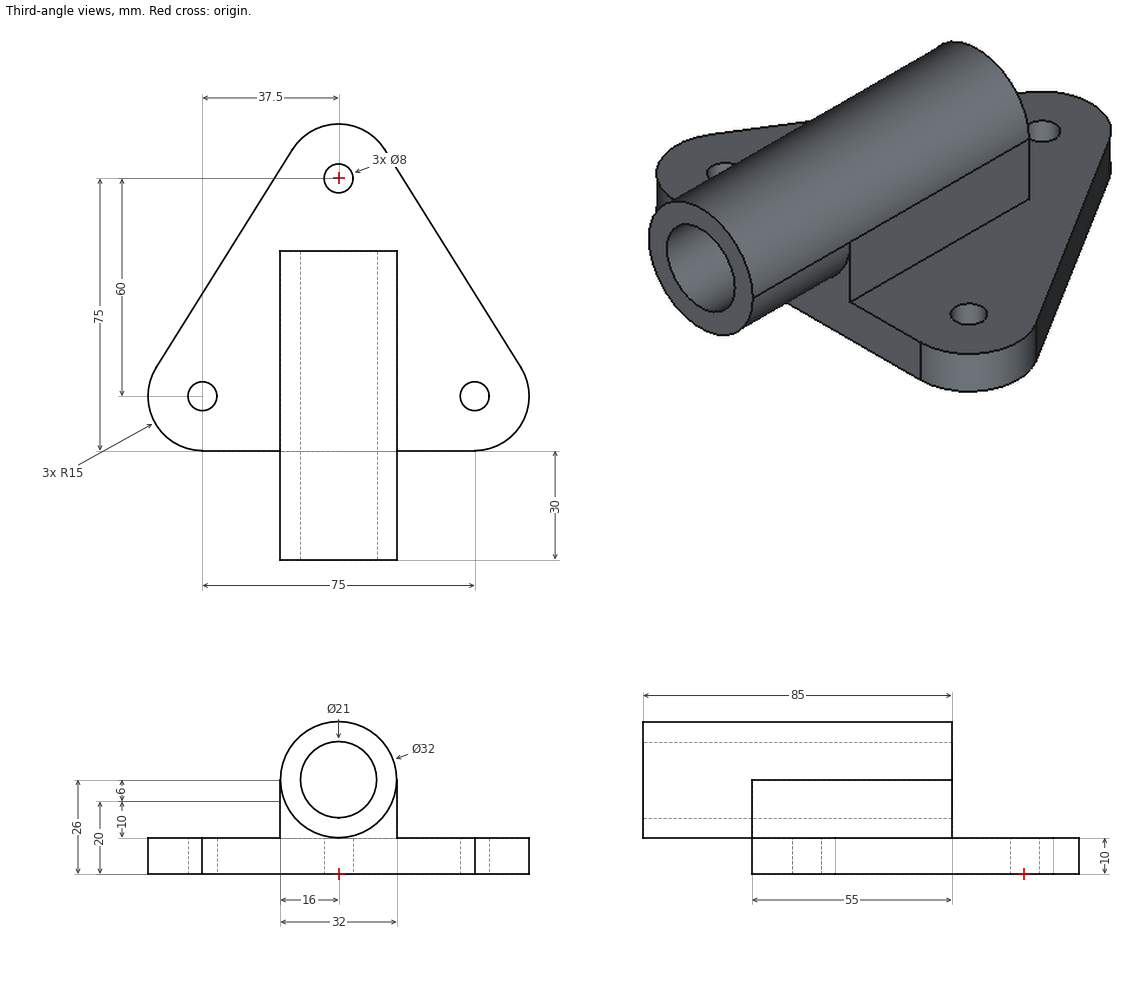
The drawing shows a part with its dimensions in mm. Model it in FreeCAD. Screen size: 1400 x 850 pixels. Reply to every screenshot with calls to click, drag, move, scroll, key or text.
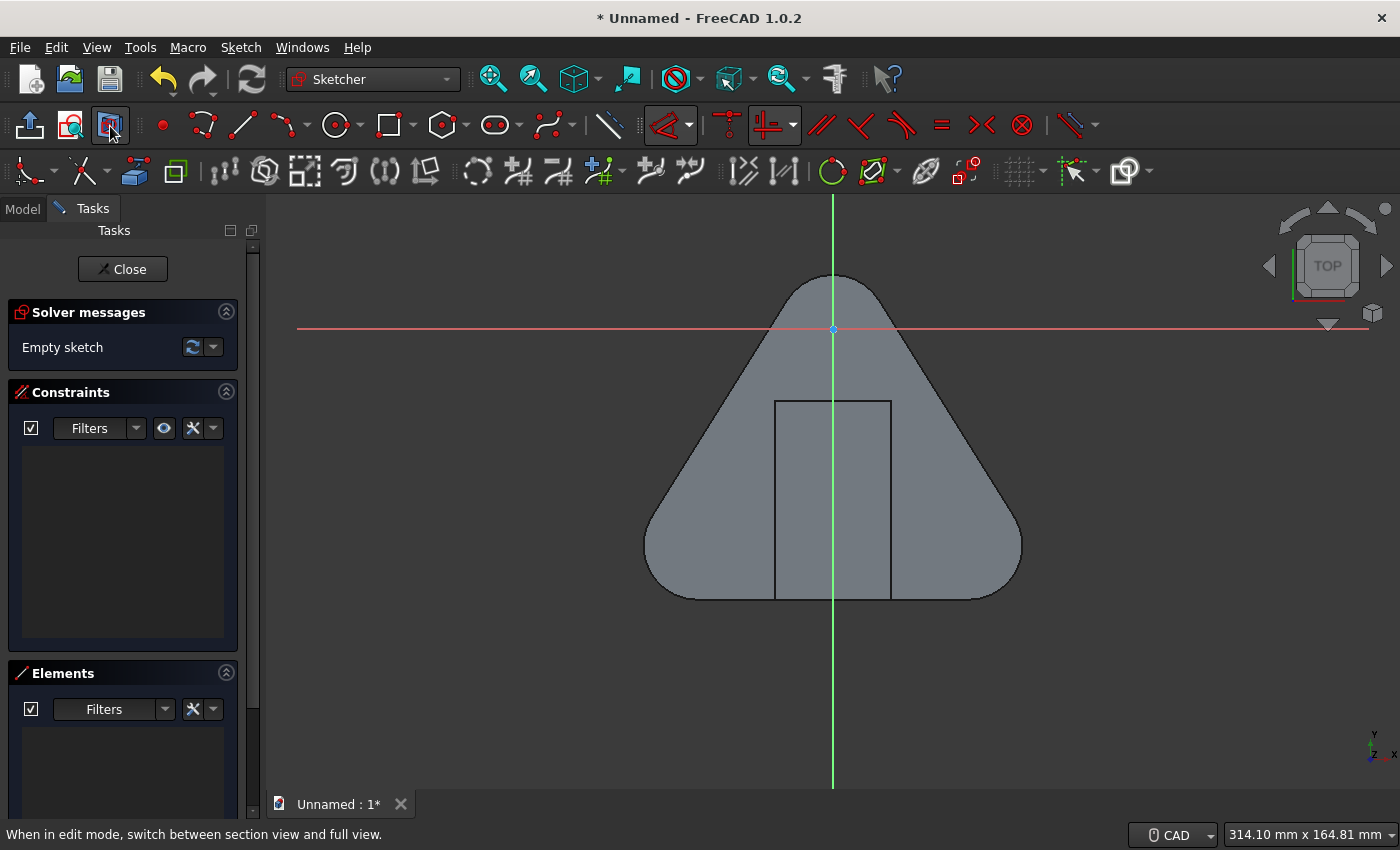
scroll(972, 327, up, 2)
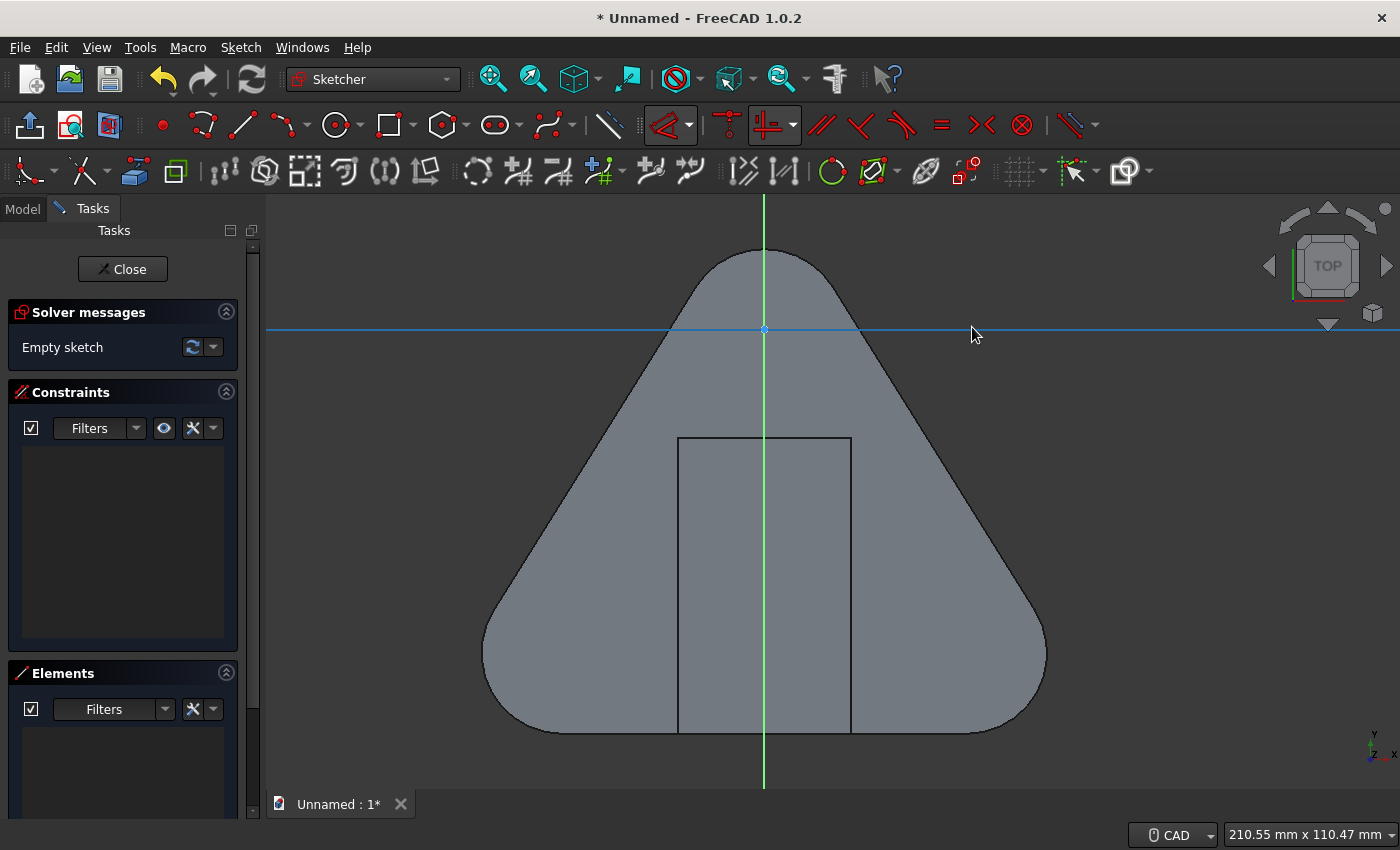
click(336, 126)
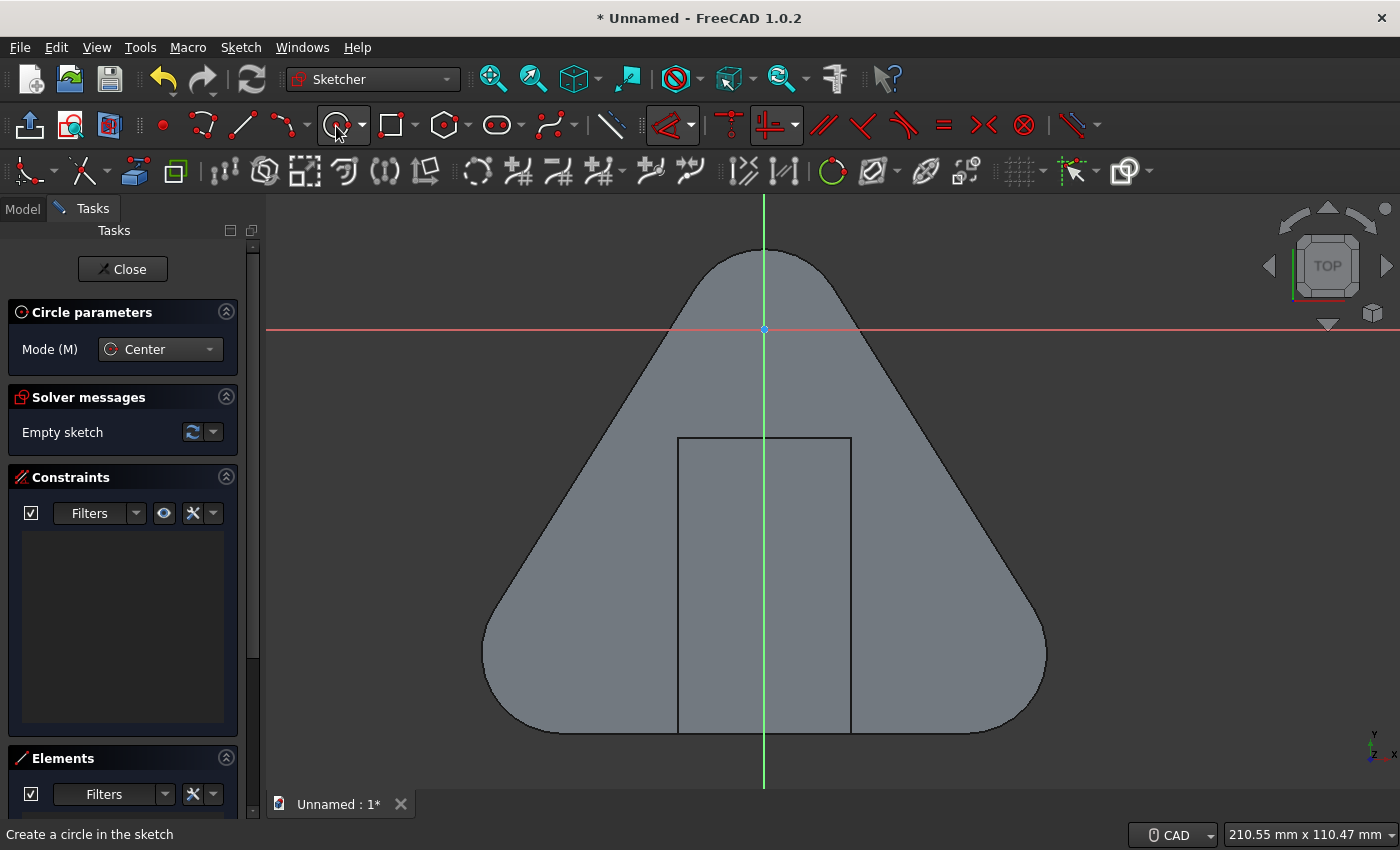
click(764, 330)
click(780, 315)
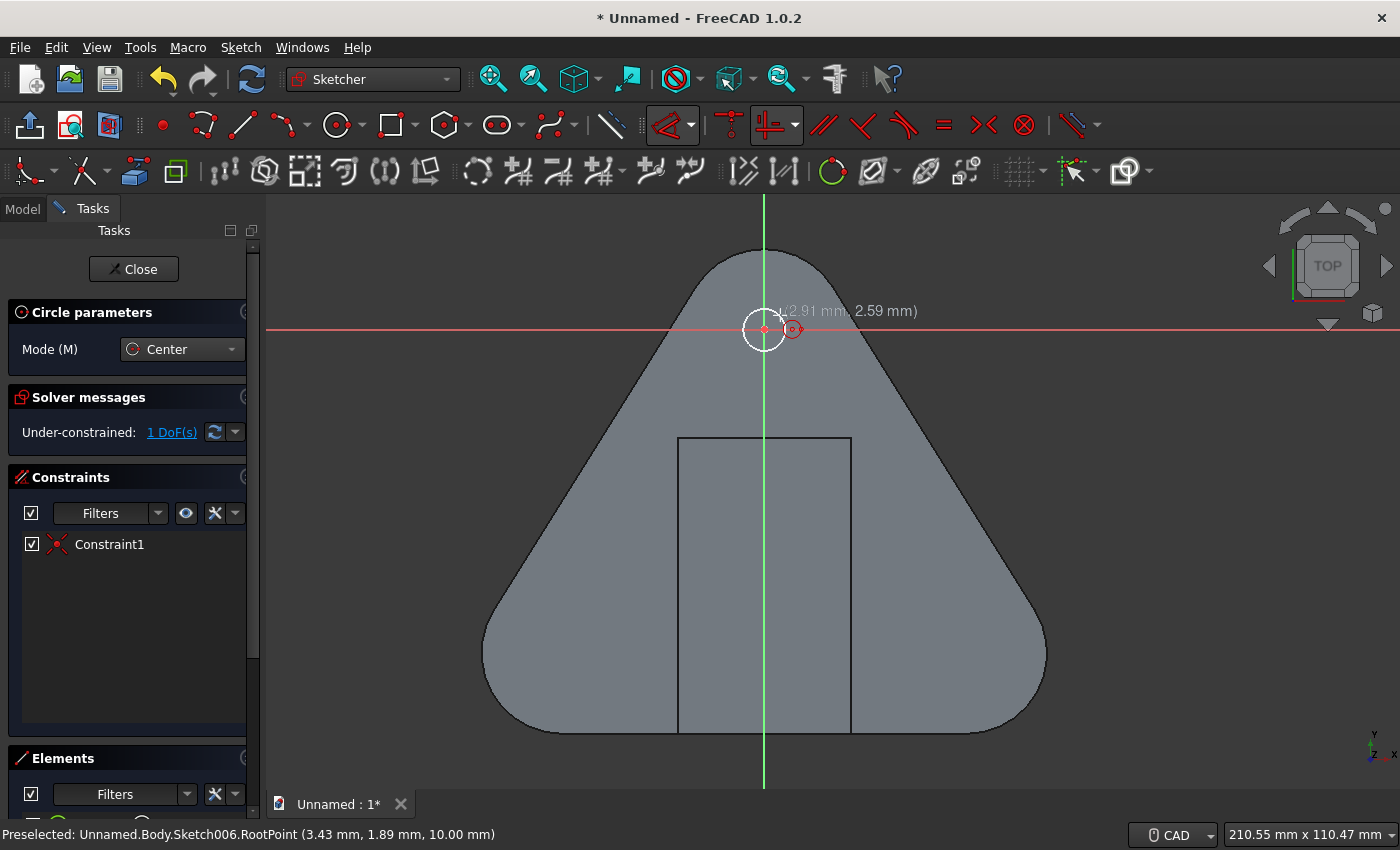
click(562, 653)
click(578, 638)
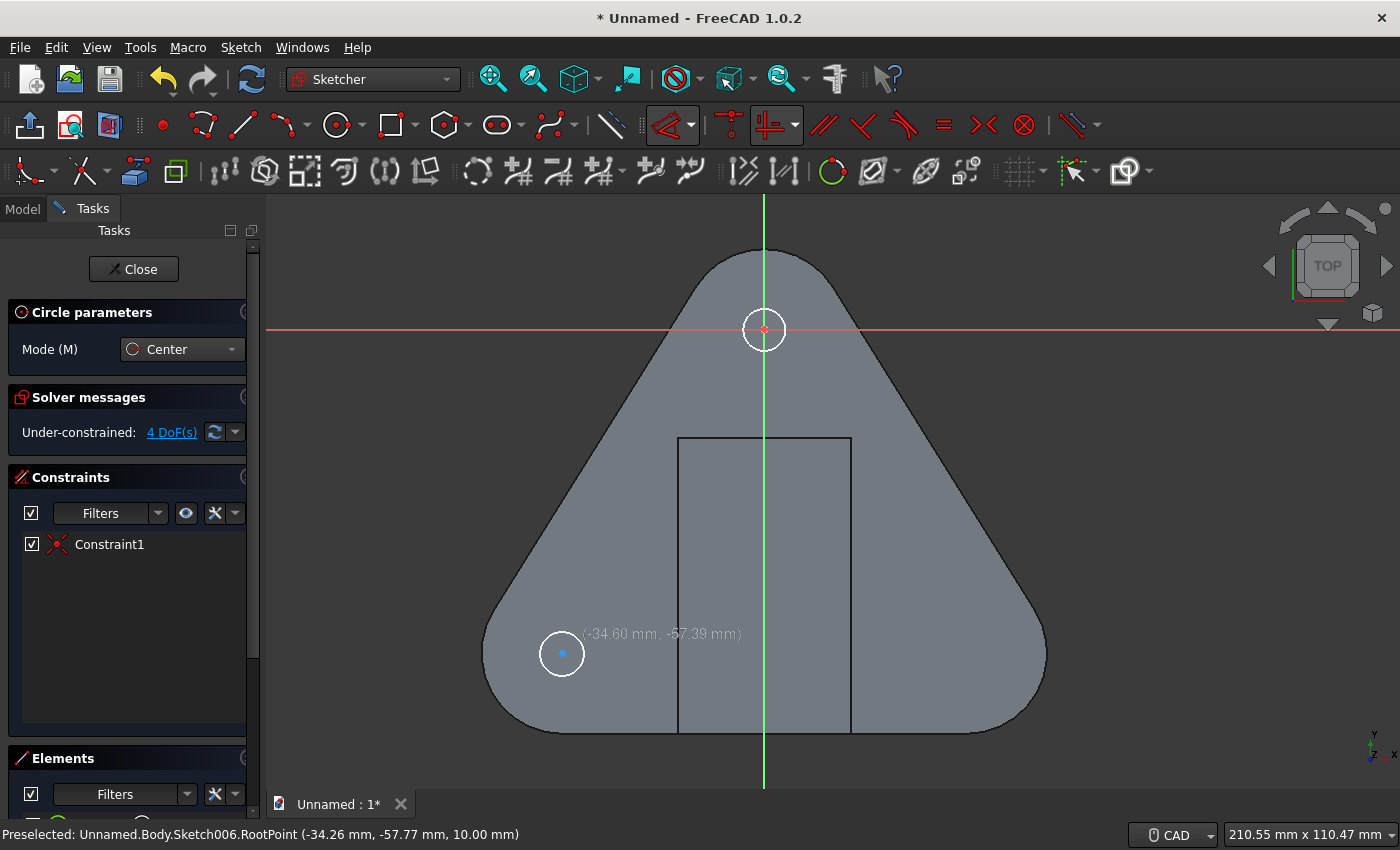
click(966, 653)
click(982, 638)
key(Escape)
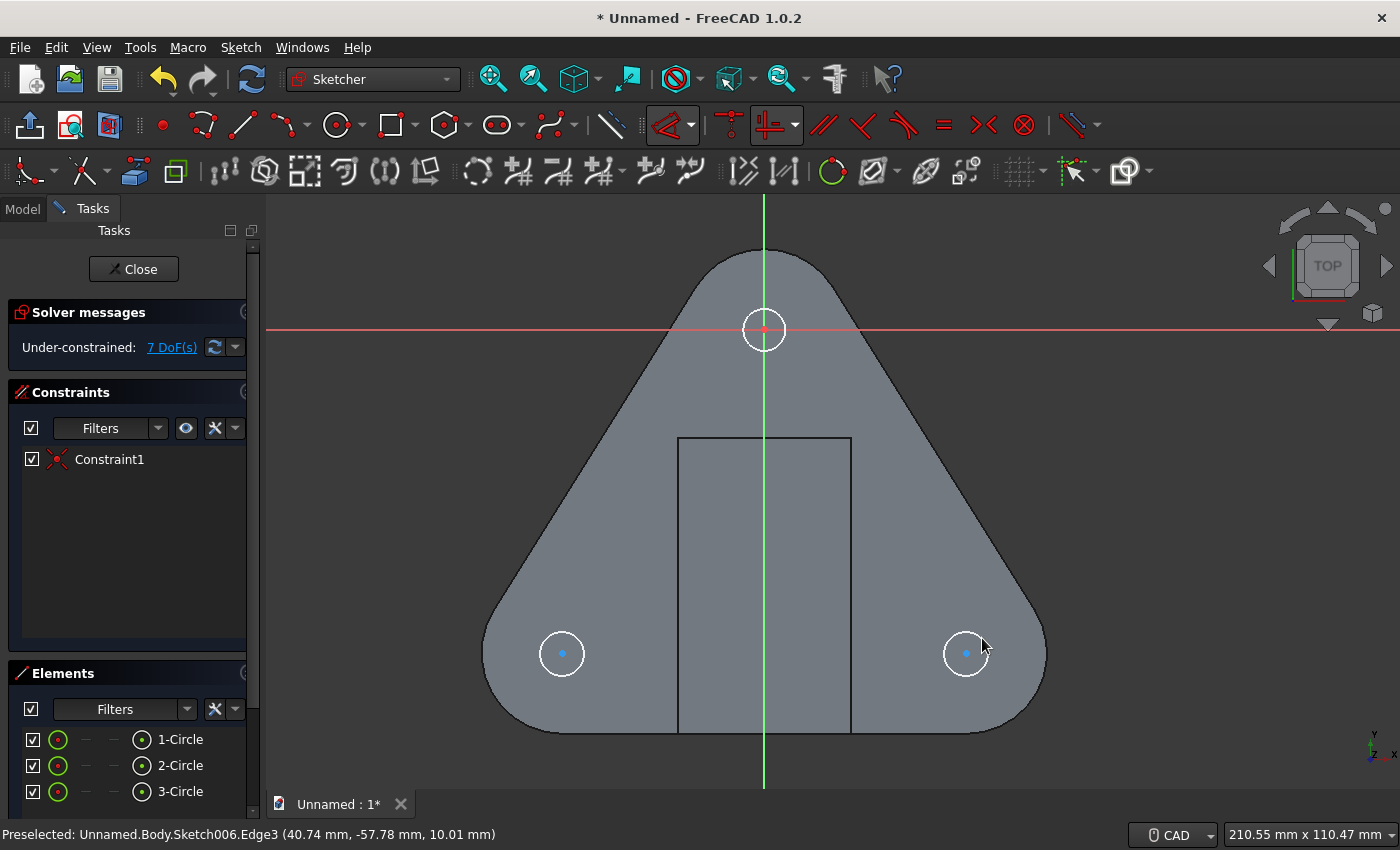
click(779, 315)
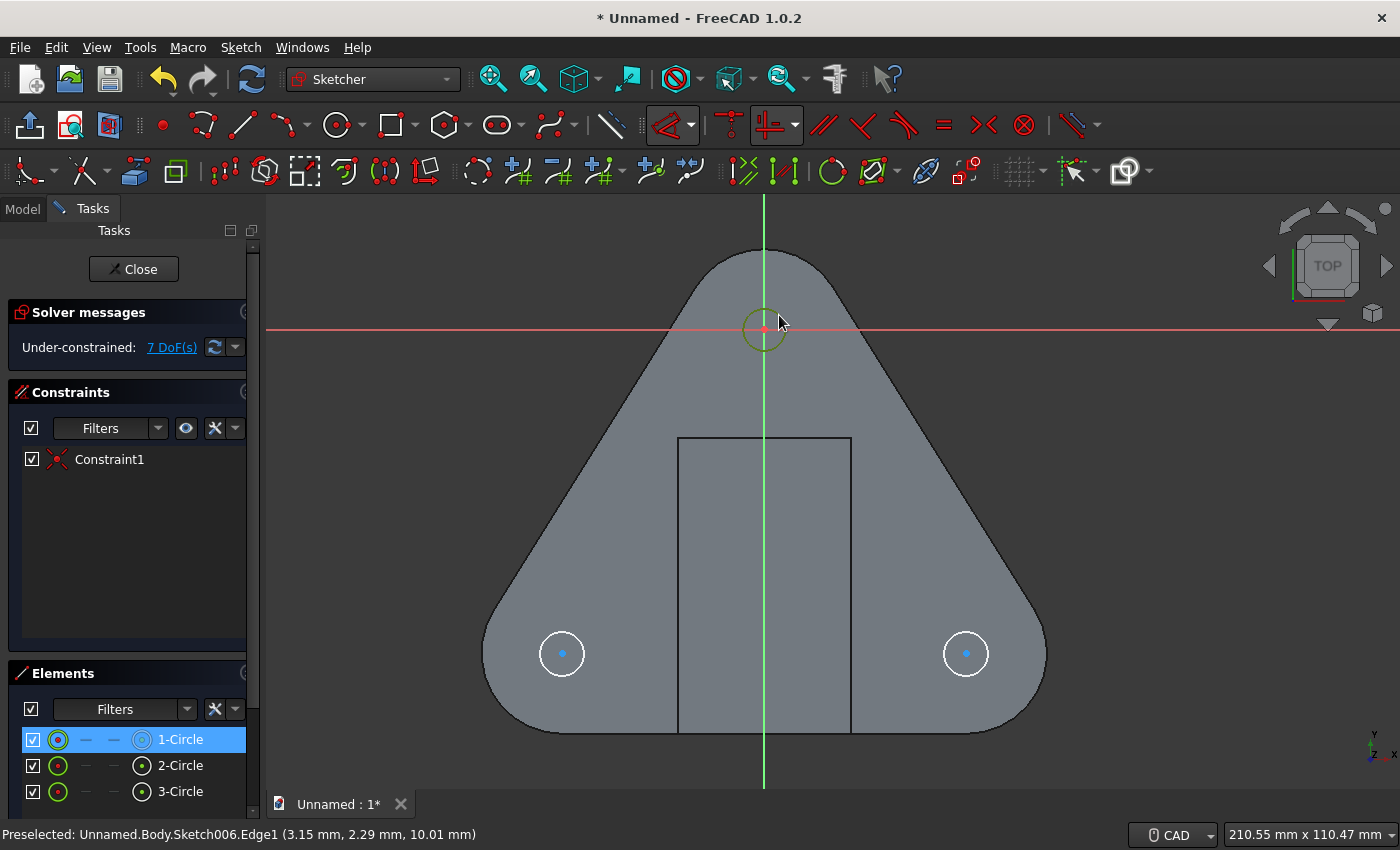
click(577, 638)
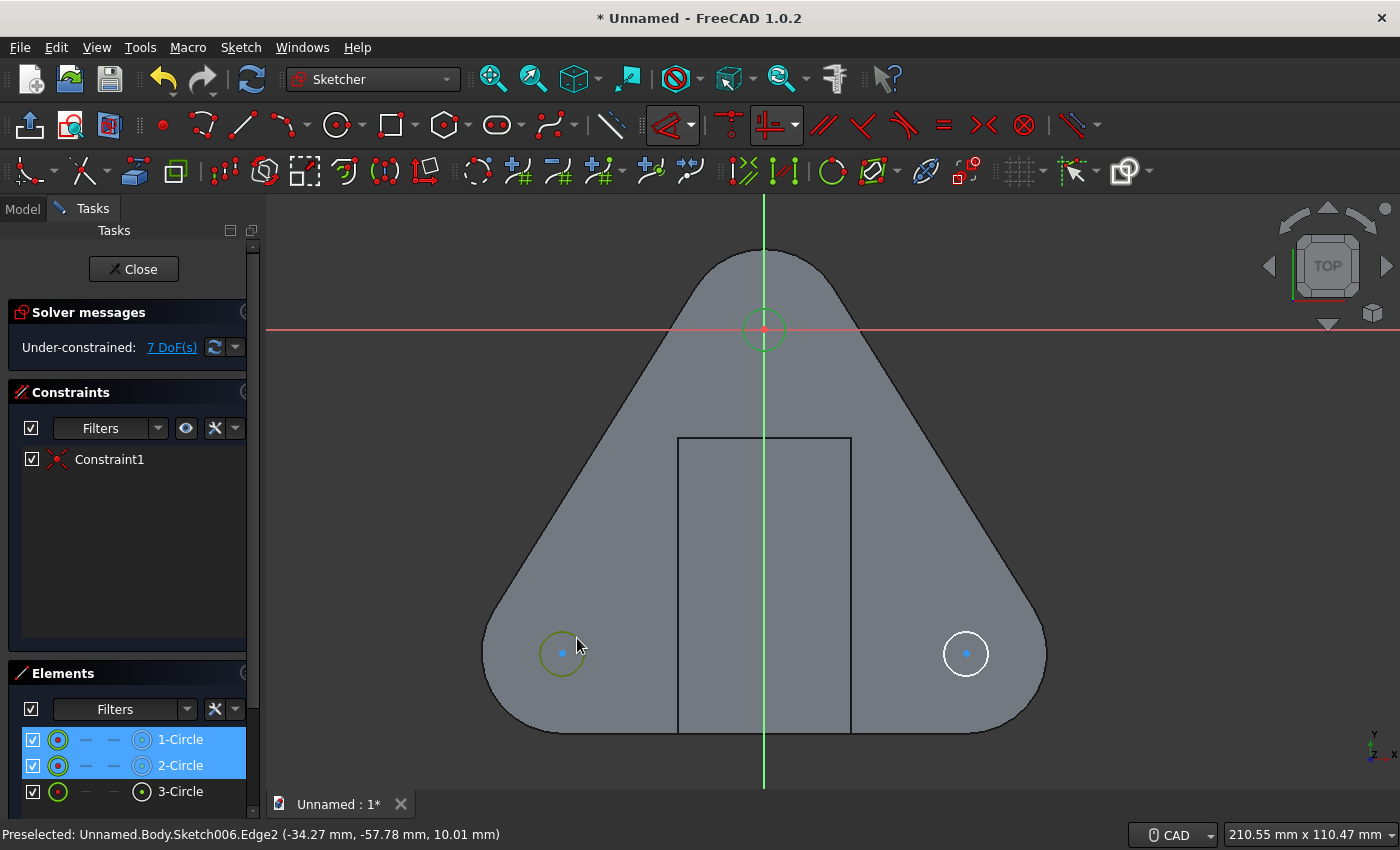
click(981, 638)